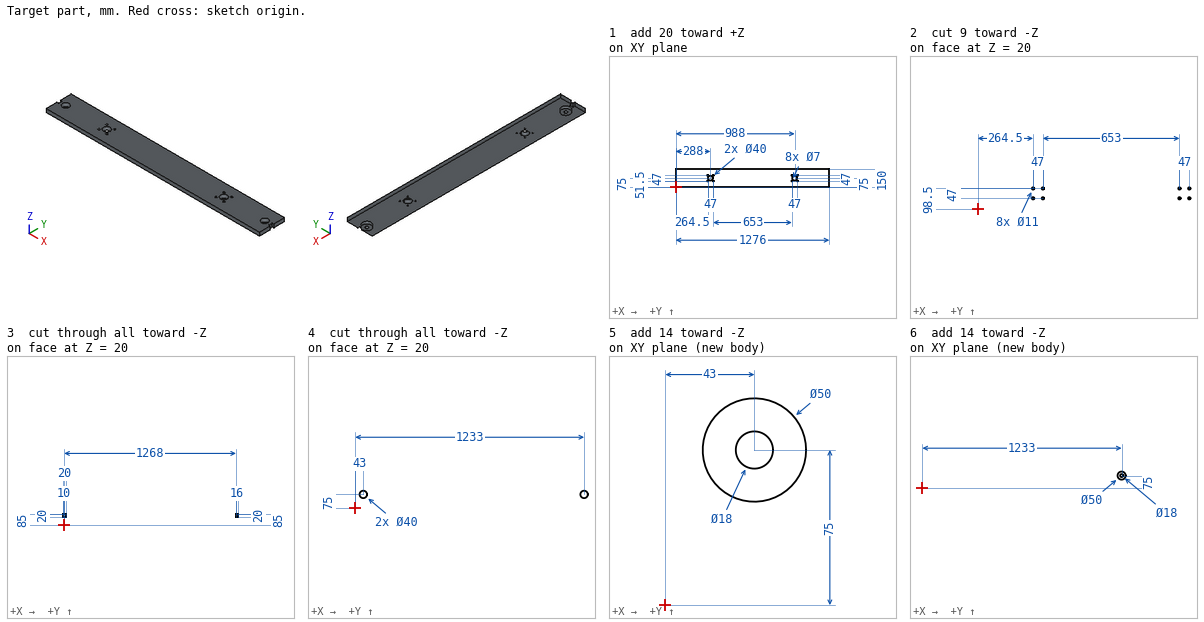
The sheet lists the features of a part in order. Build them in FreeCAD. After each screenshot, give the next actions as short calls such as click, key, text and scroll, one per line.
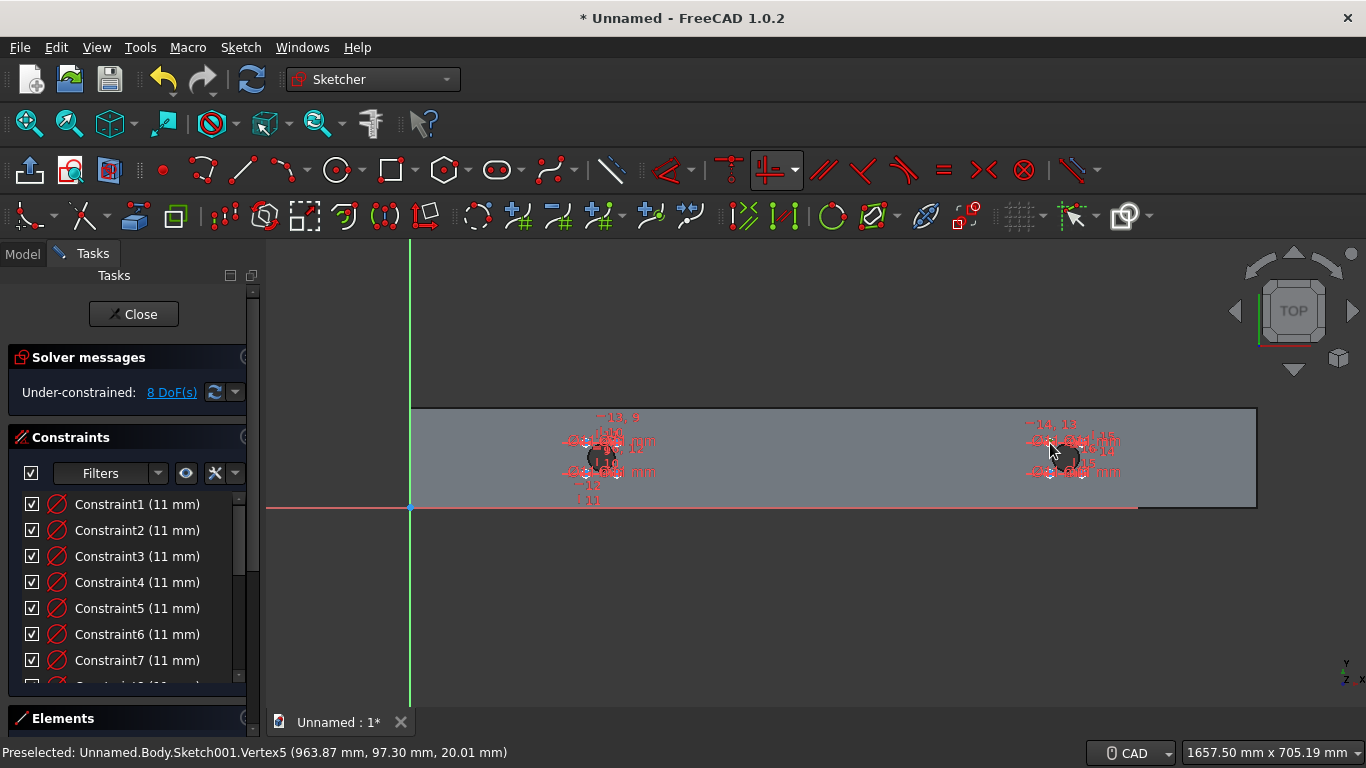
click(1050, 474)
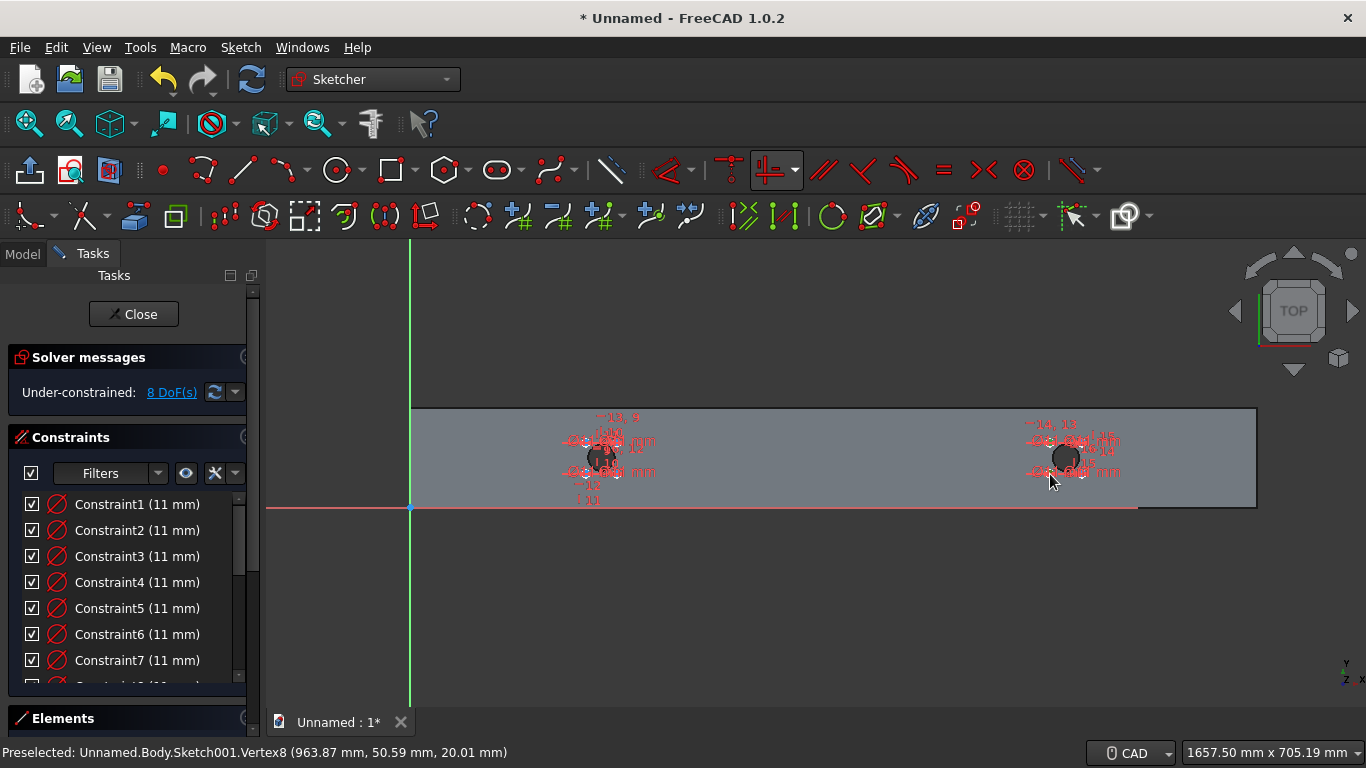
click(798, 170)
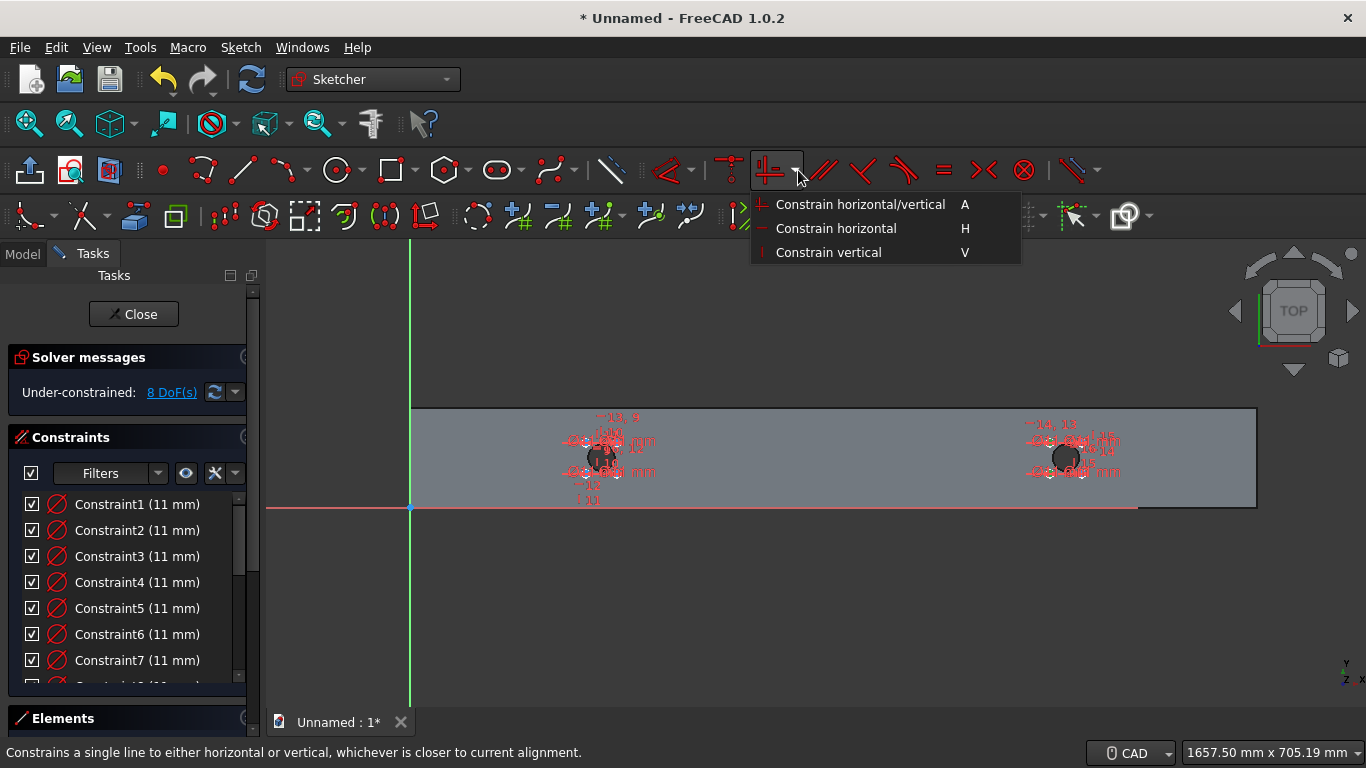
click(886, 252)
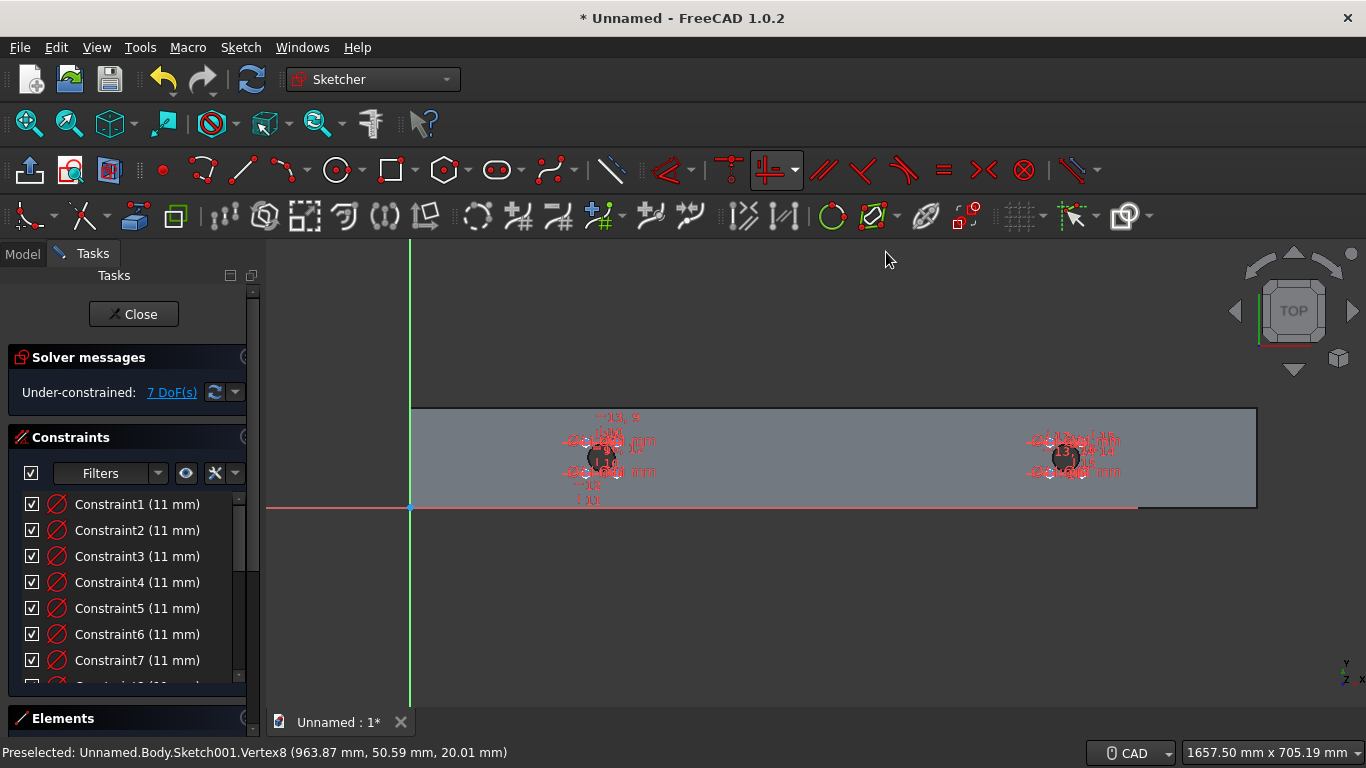
click(1084, 476)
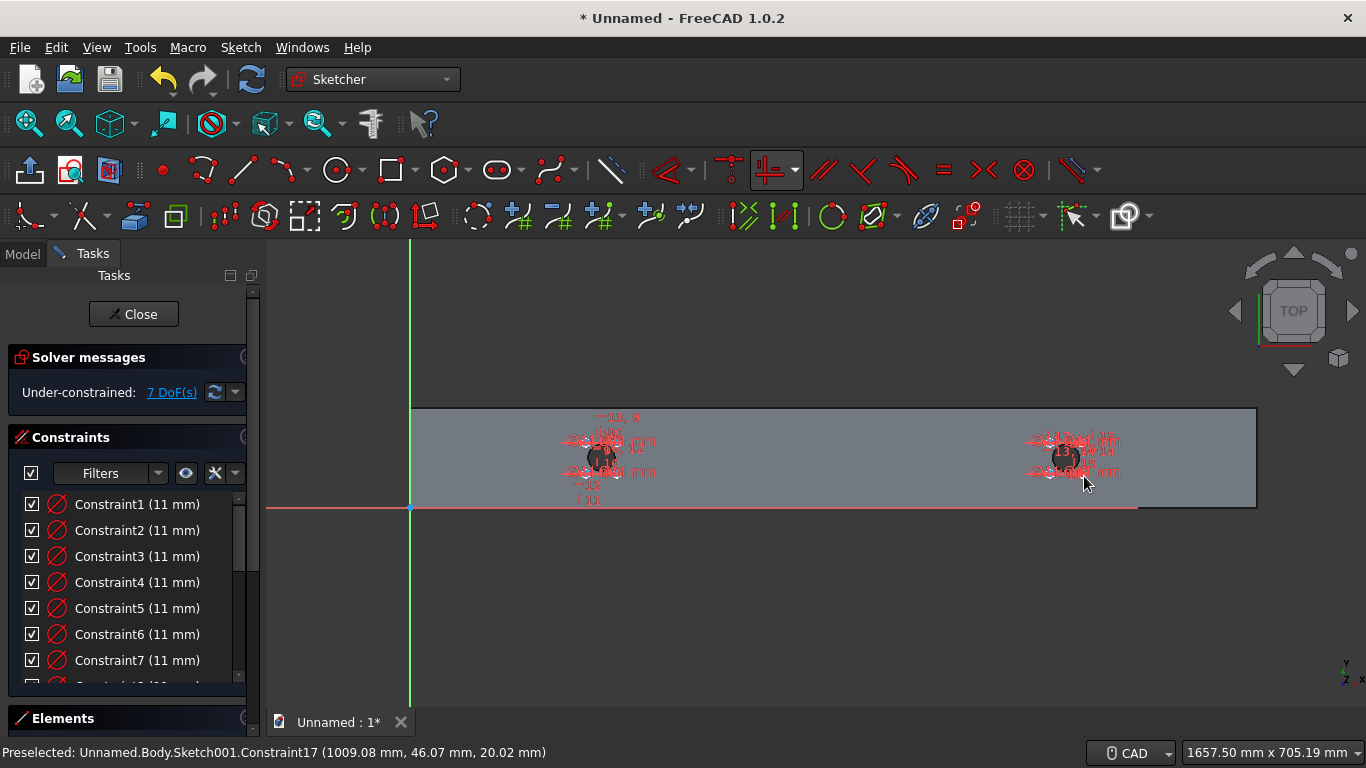
click(1050, 474)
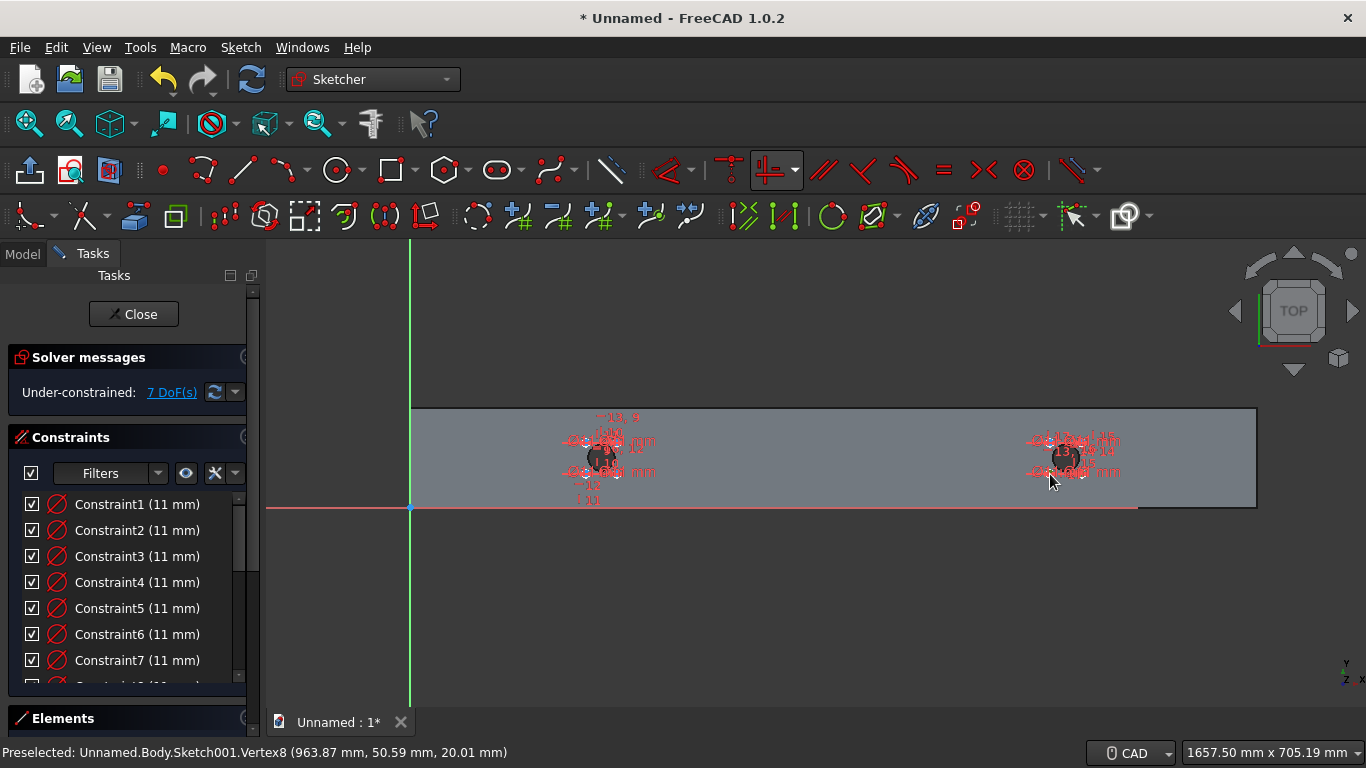
click(798, 170)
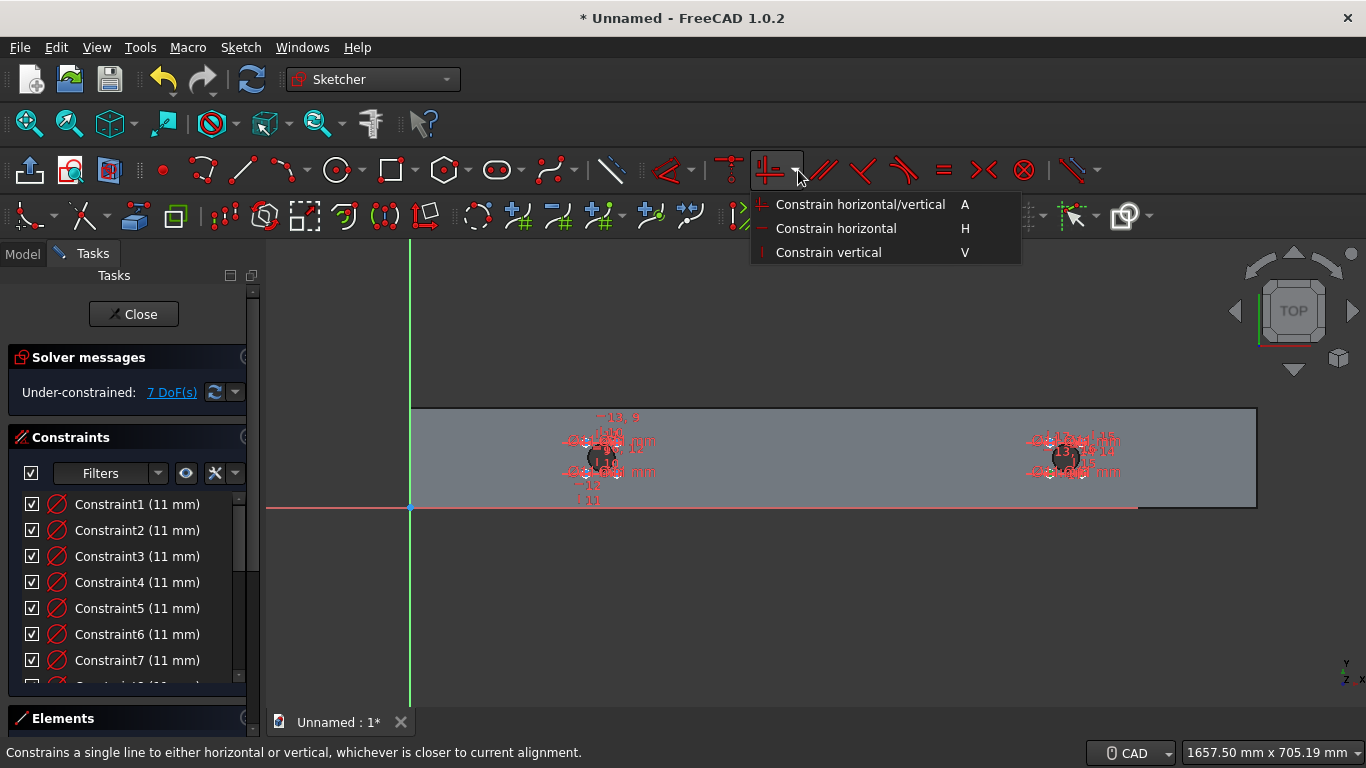
click(886, 228)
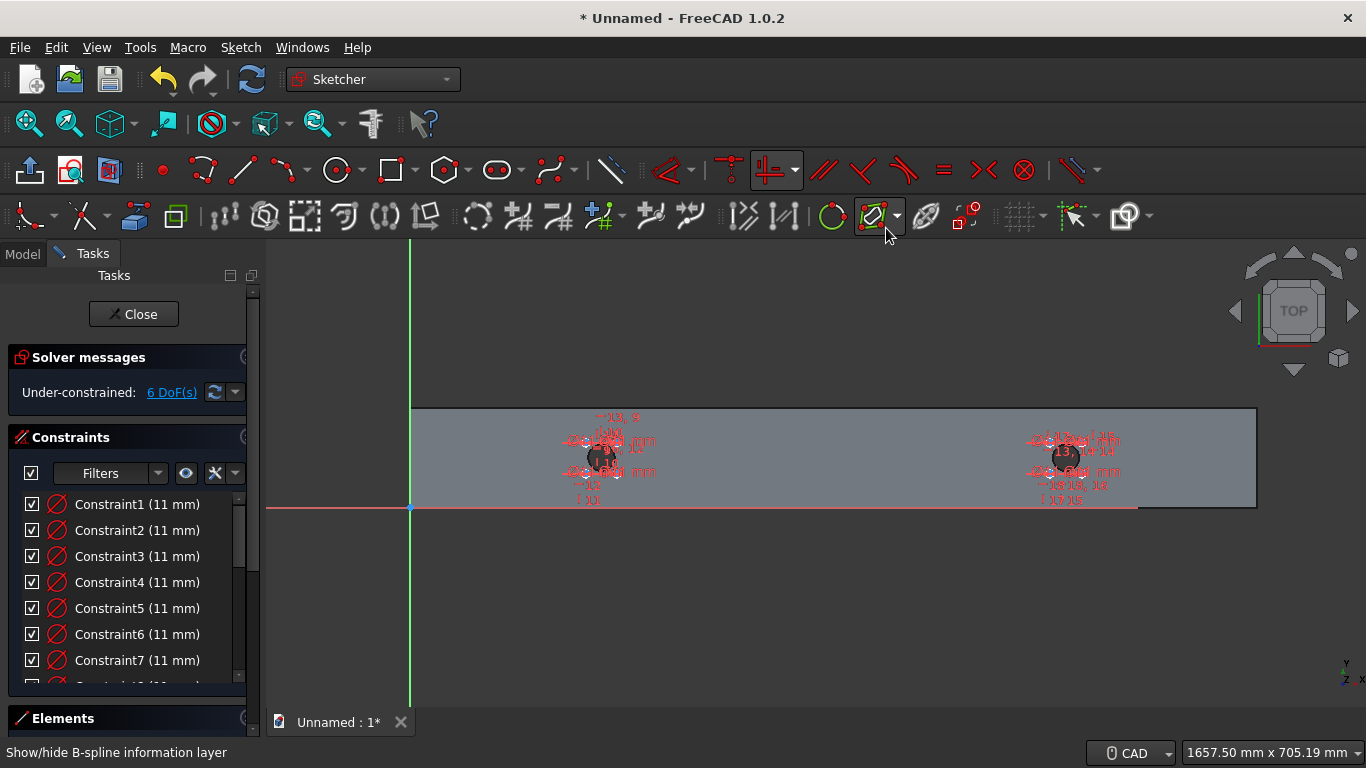
click(666, 170)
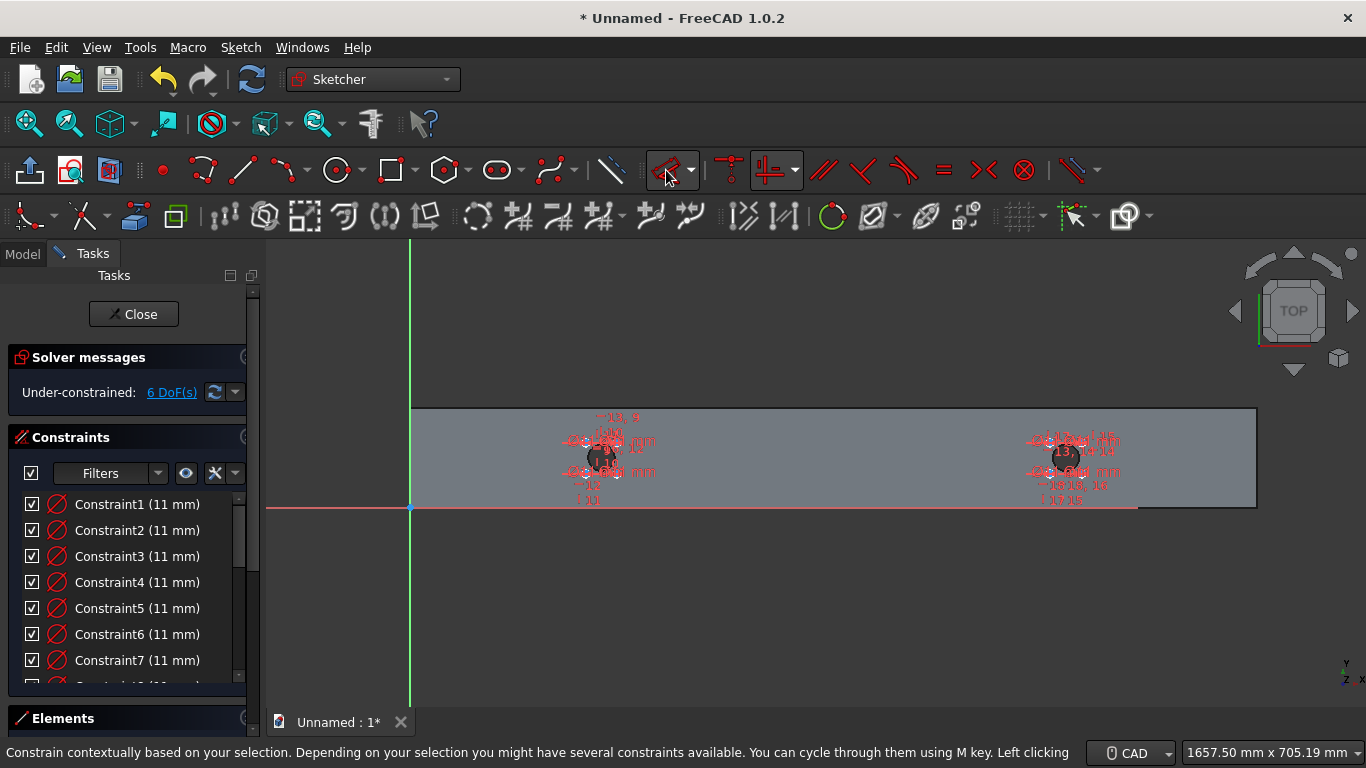
scroll(586, 443, up, 2)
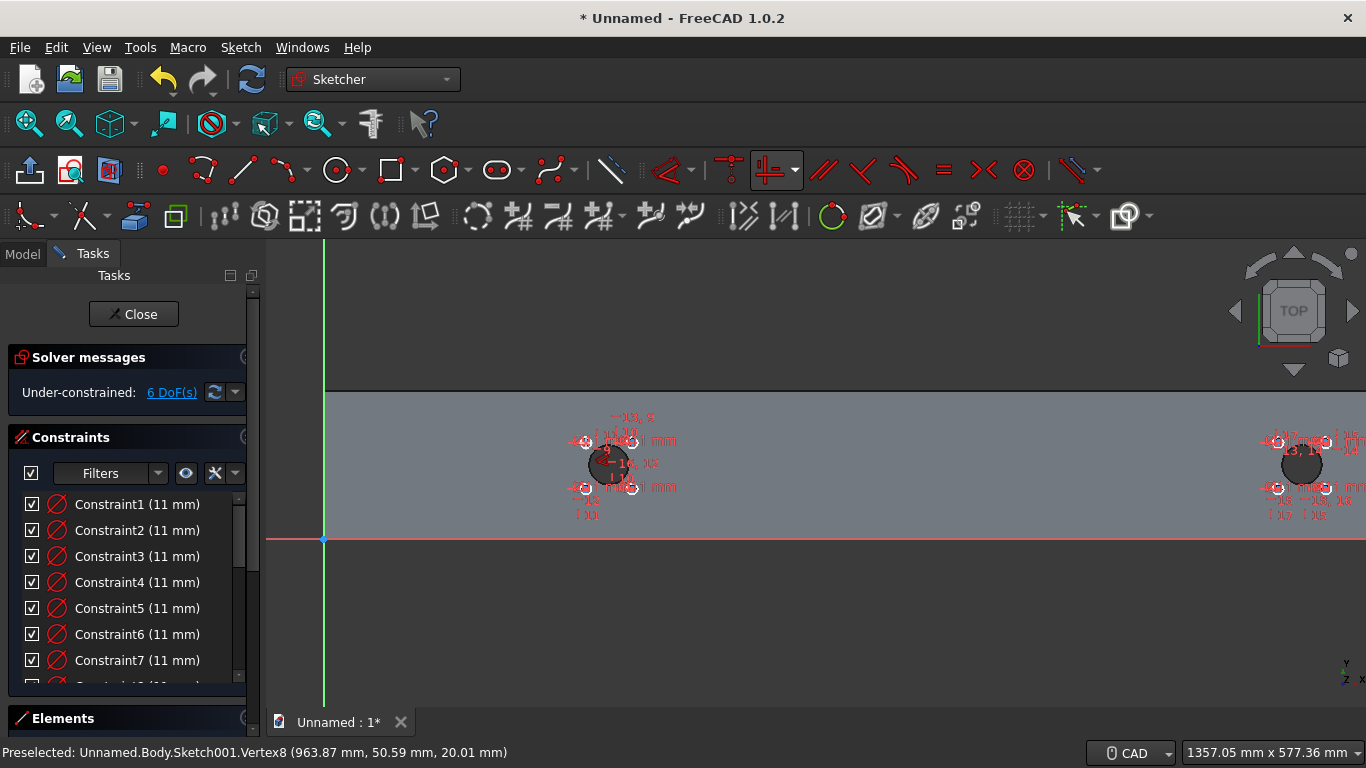
click(586, 443)